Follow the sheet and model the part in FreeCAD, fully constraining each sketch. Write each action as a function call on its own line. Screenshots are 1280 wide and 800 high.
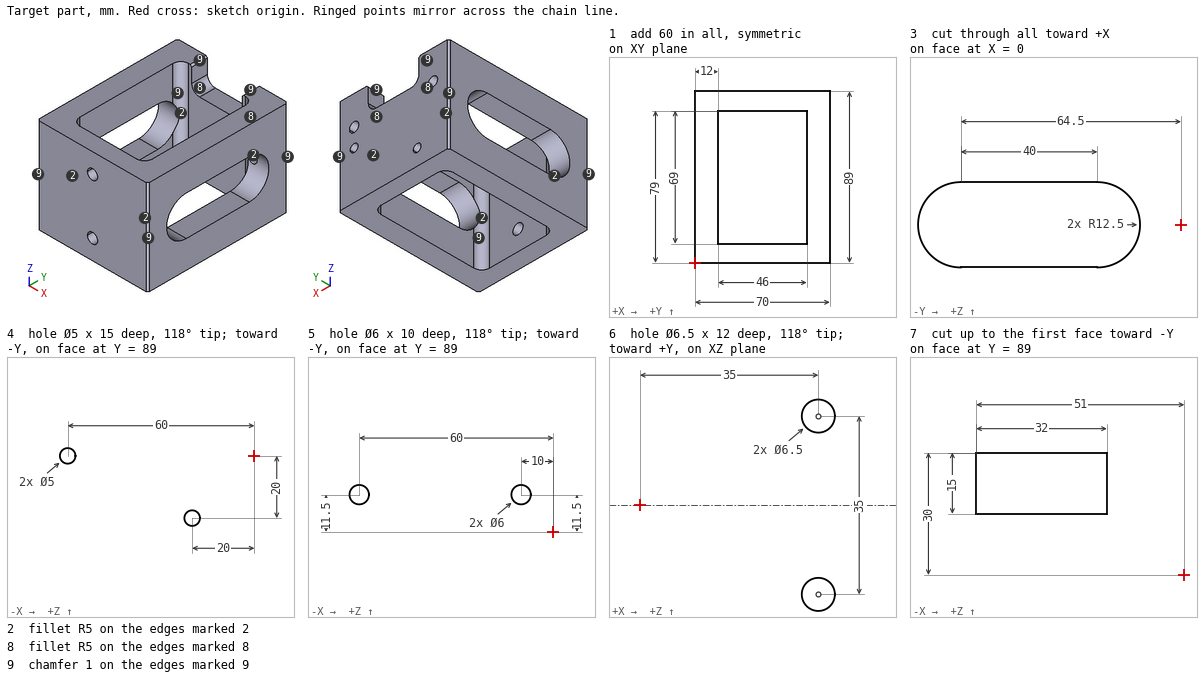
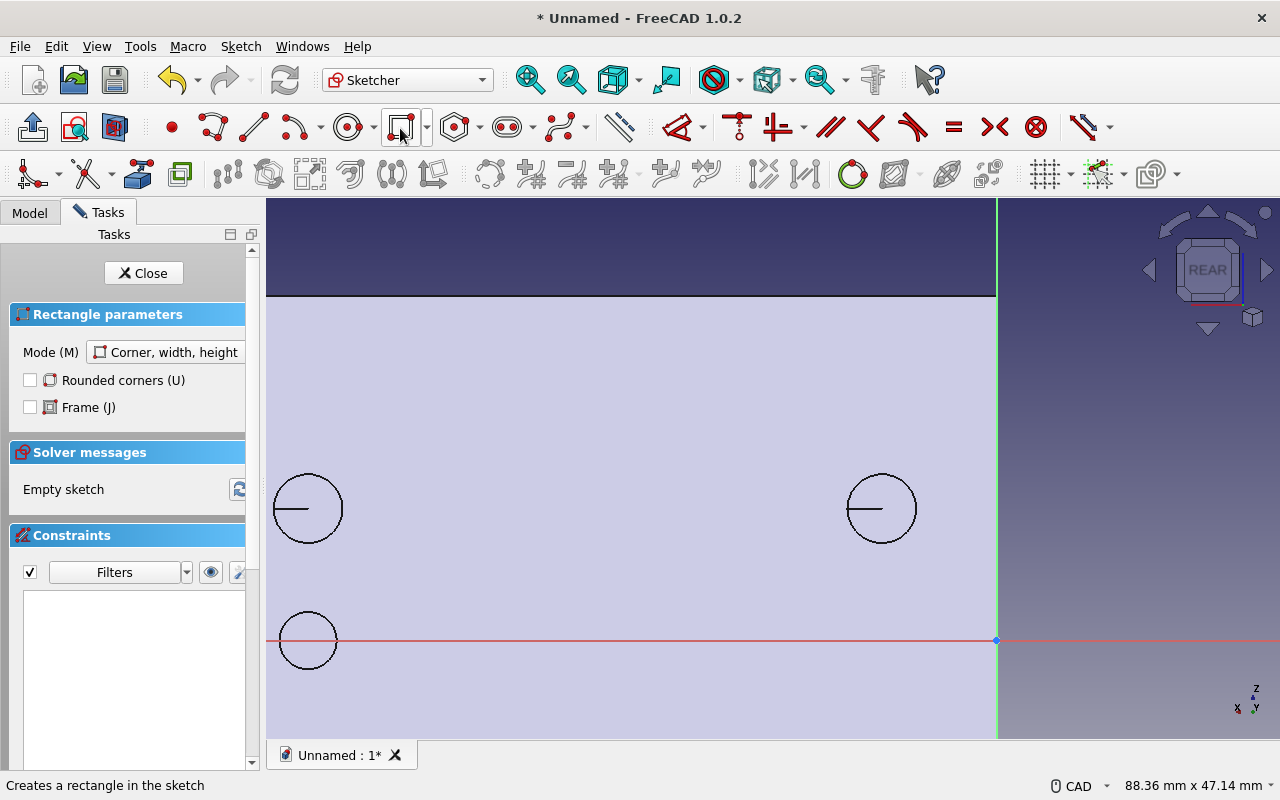
click(411, 296)
click(779, 469)
key(Escape)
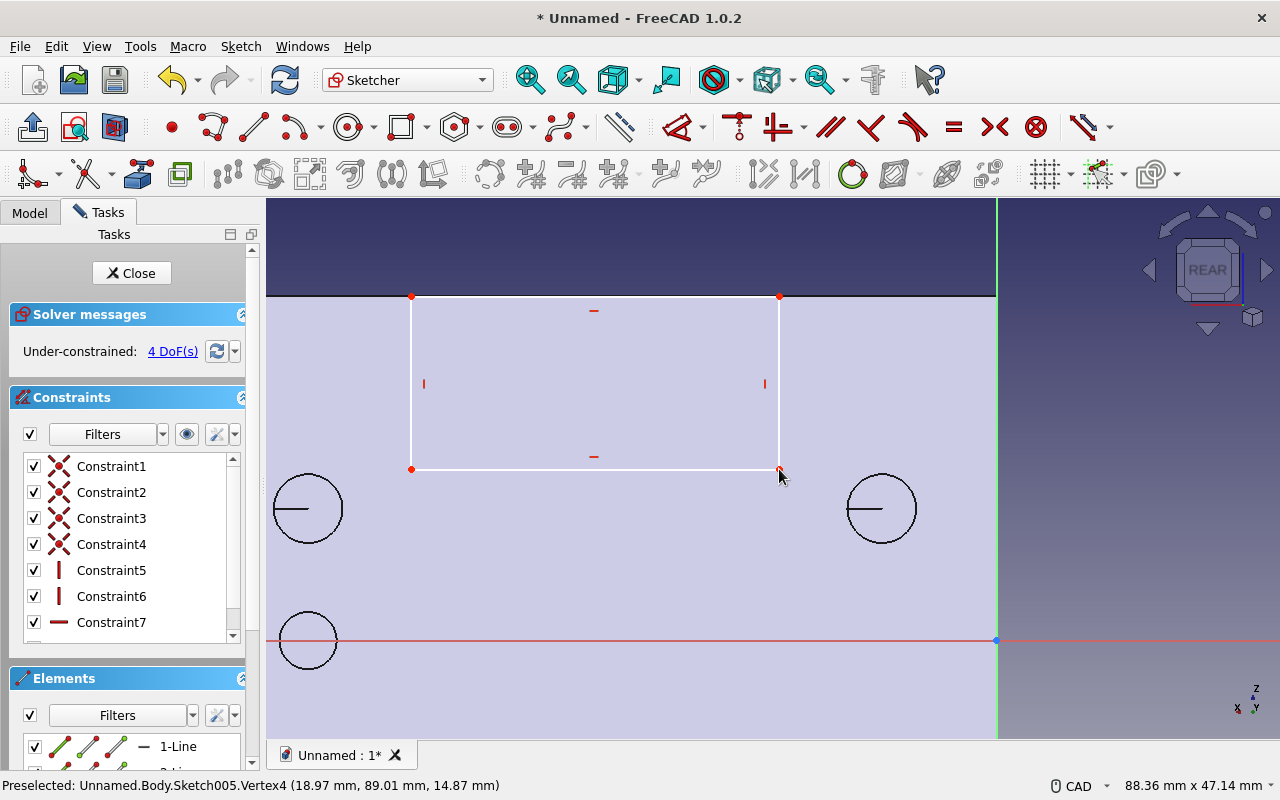
click(676, 128)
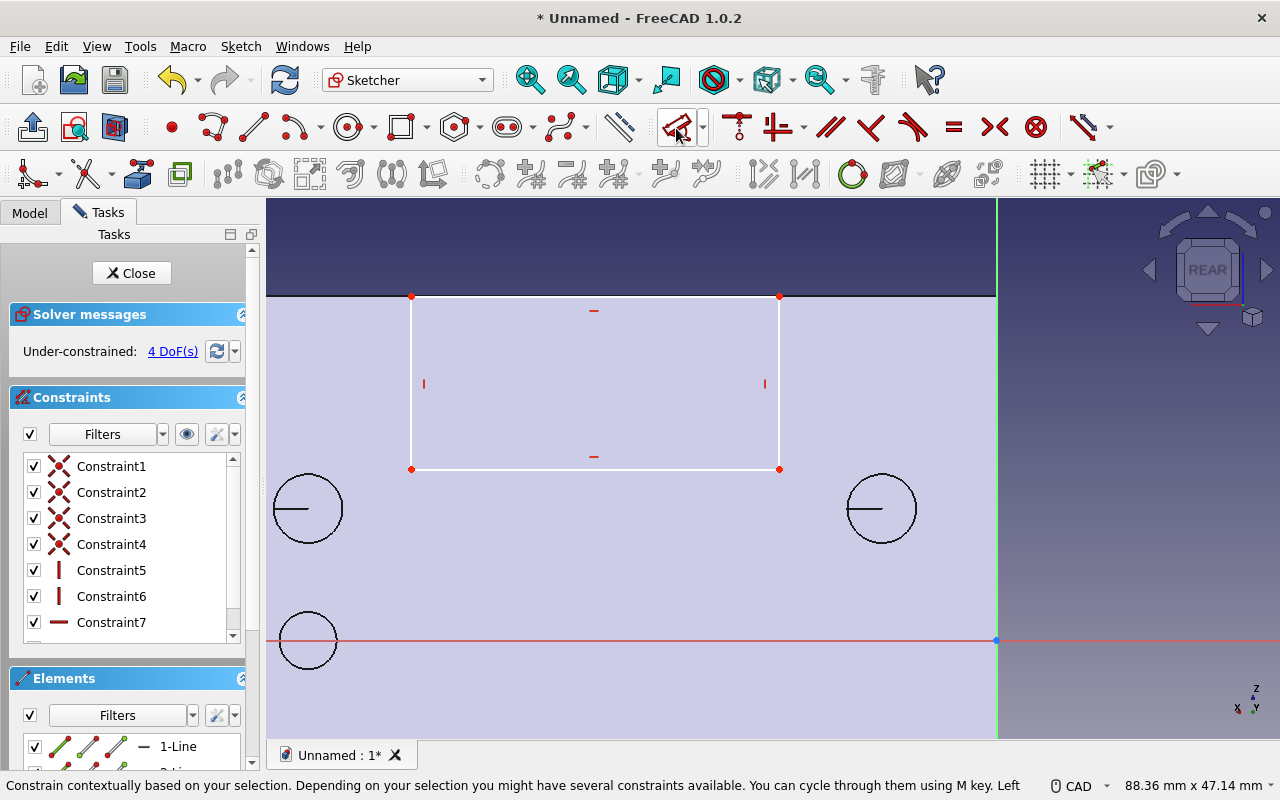
click(411, 349)
click(377, 383)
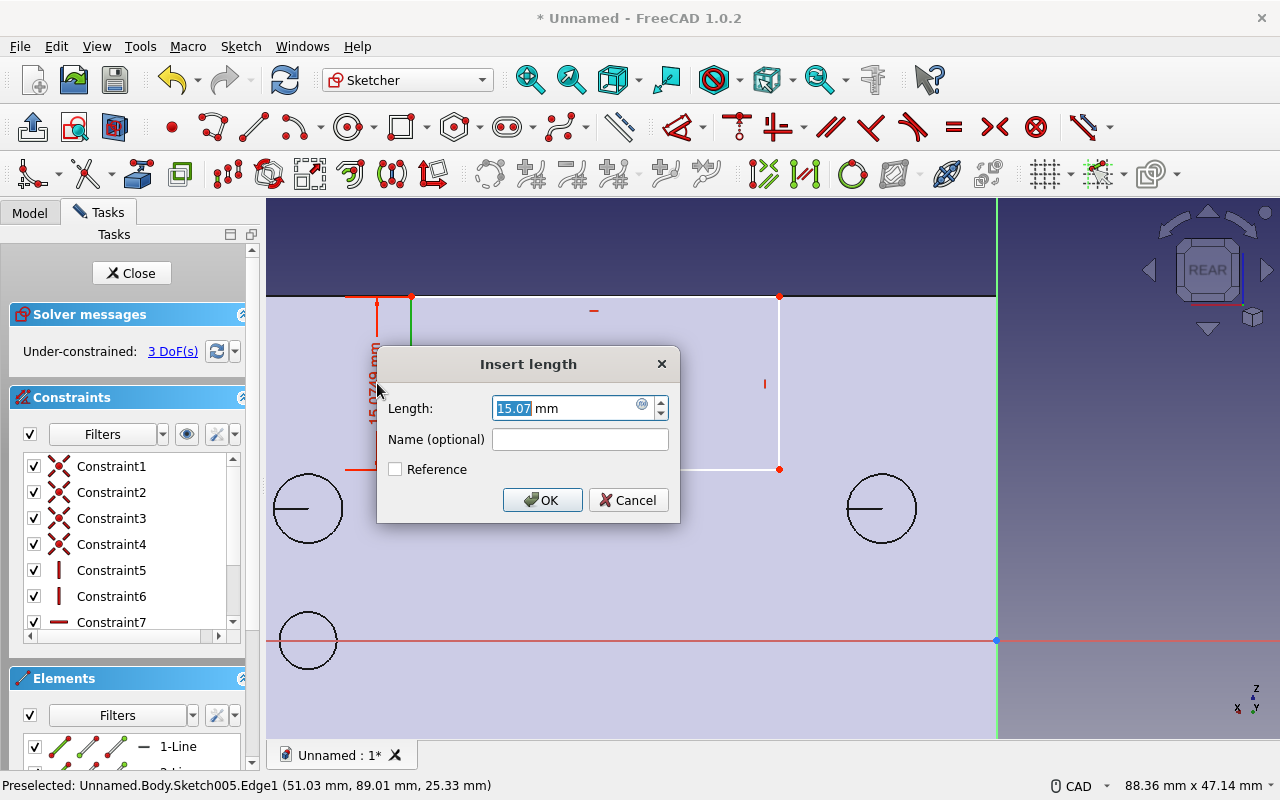
text(15)
key(Return)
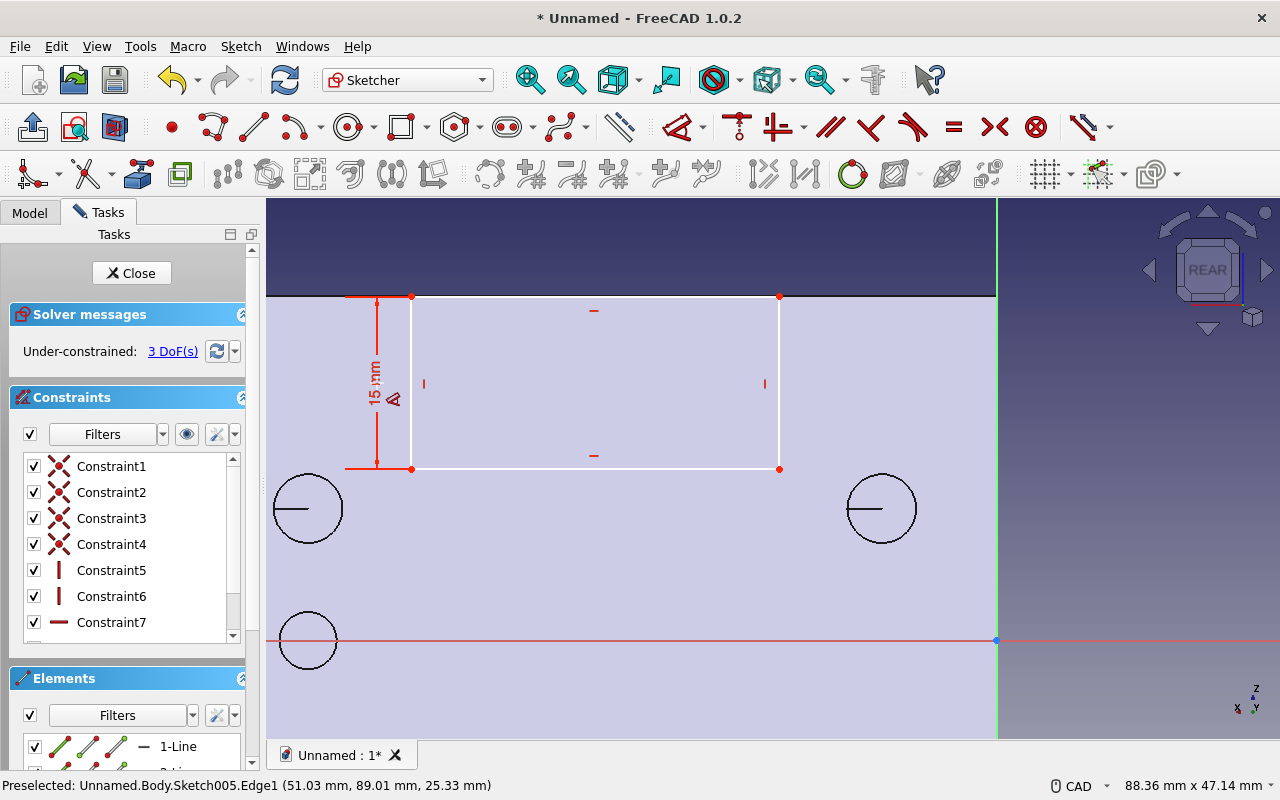
click(521, 469)
click(595, 503)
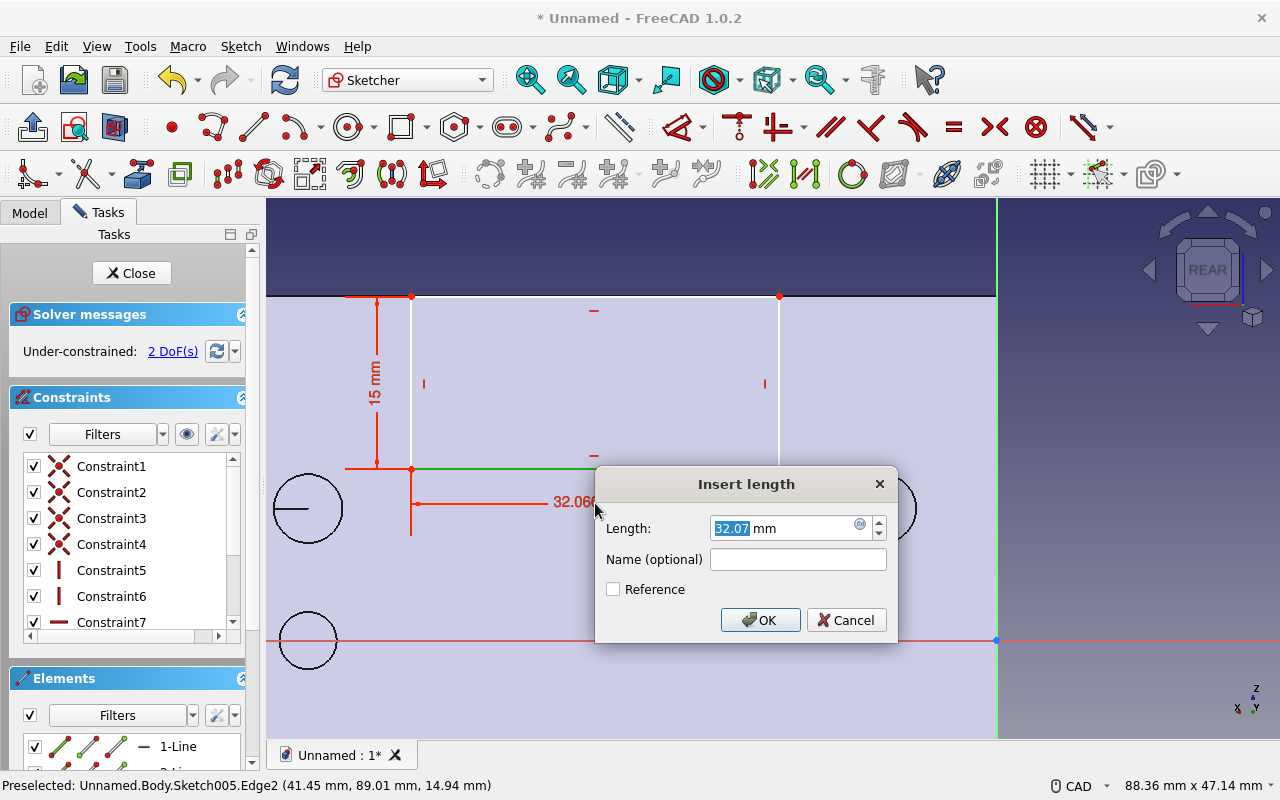
text(32)
key(Return)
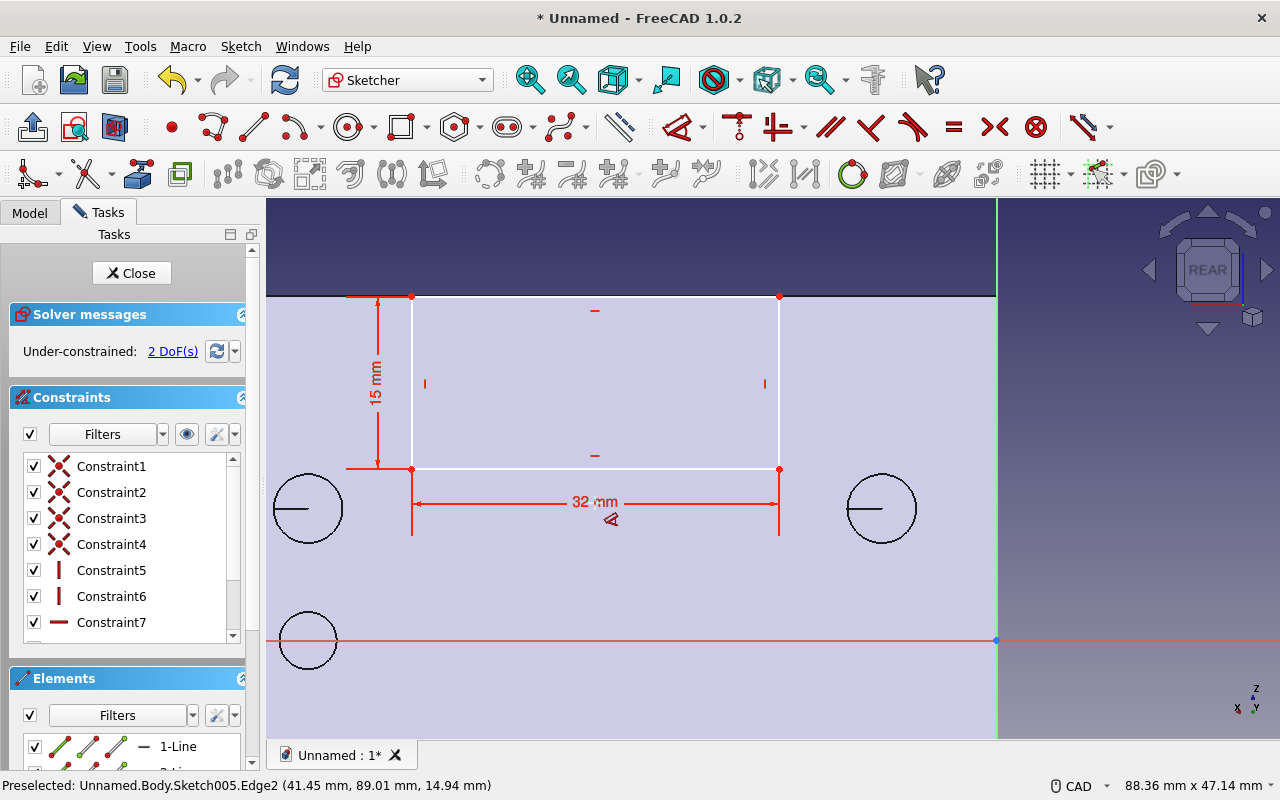
click(412, 297)
click(704, 675)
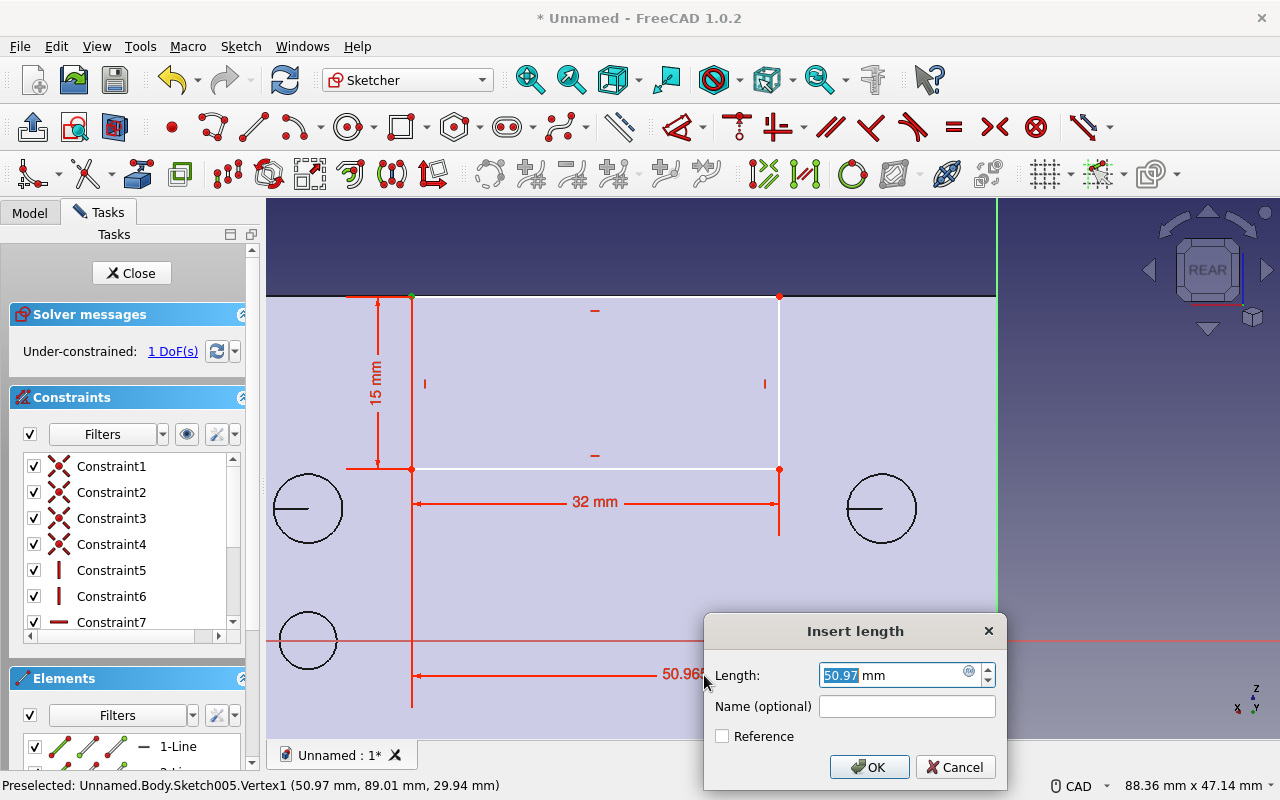
text(51)
key(Return)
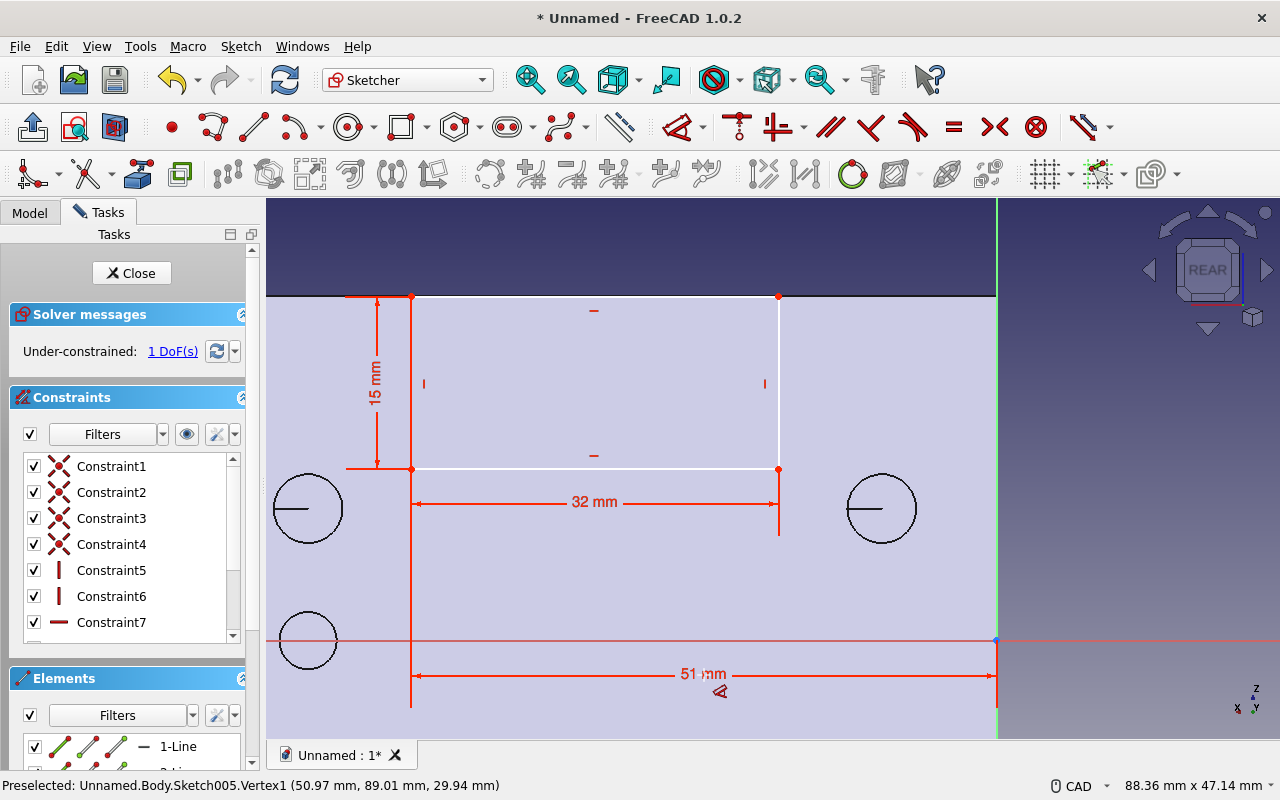
click(411, 297)
click(1031, 469)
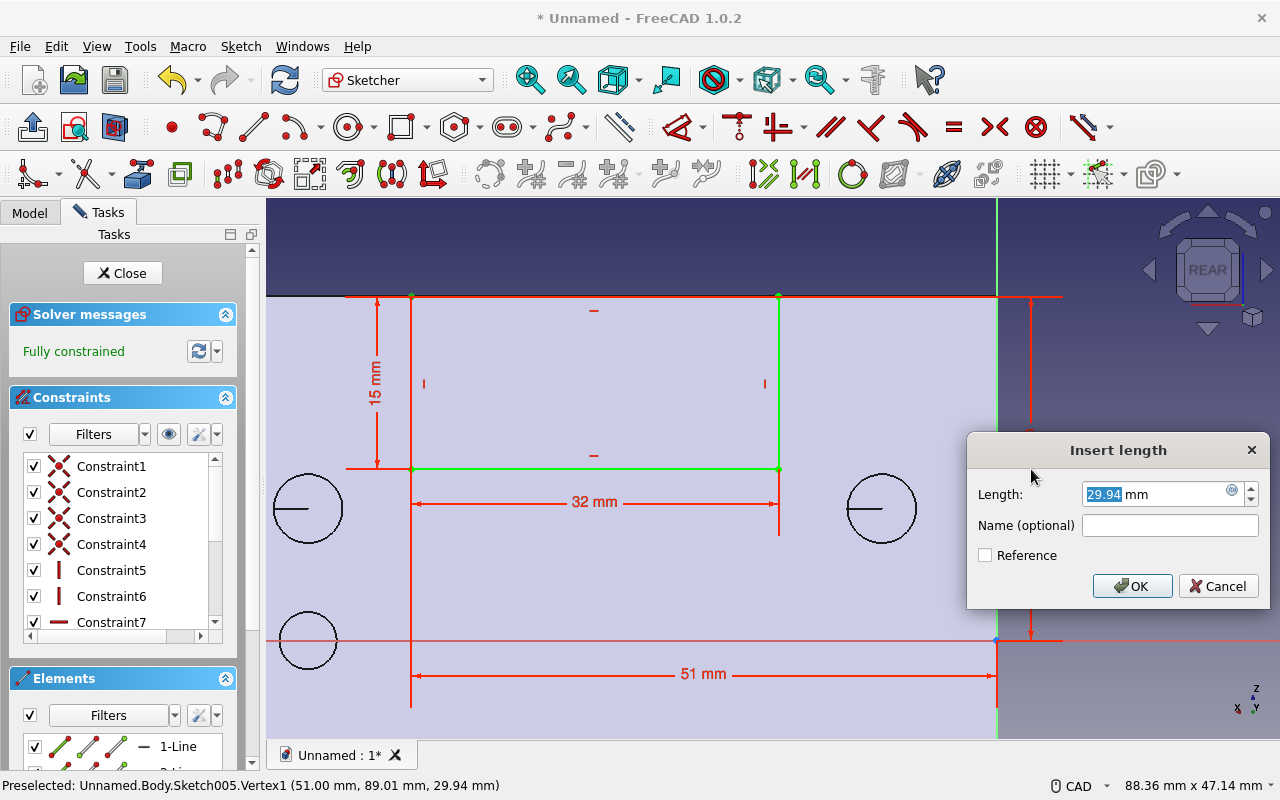
text(30)
key(Return)
key(Escape)